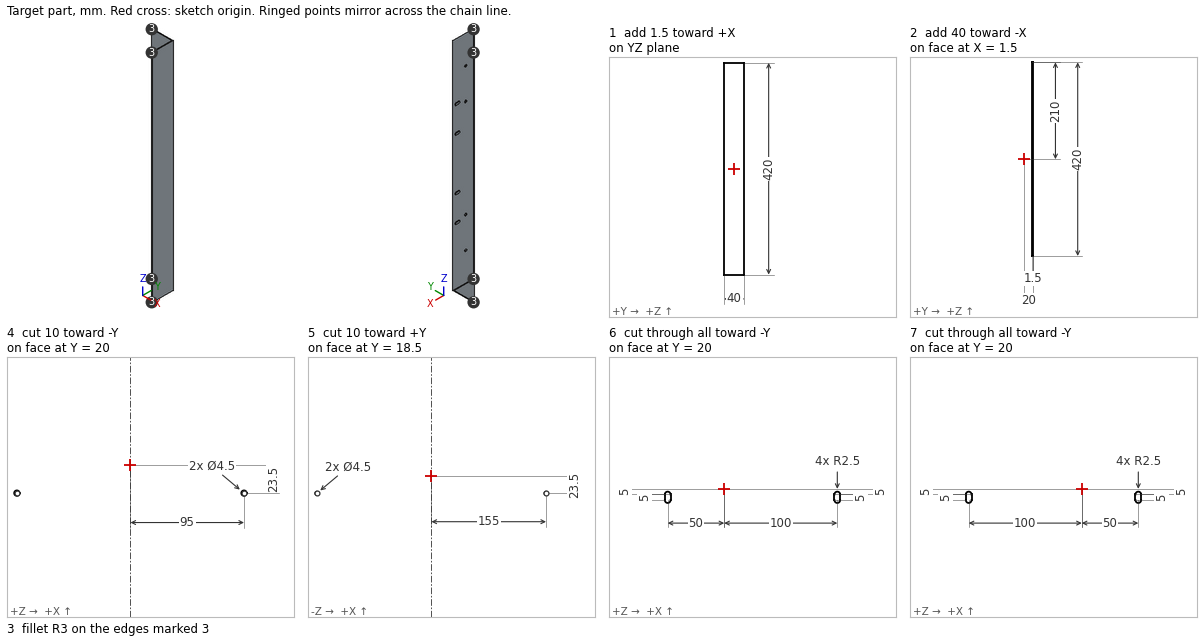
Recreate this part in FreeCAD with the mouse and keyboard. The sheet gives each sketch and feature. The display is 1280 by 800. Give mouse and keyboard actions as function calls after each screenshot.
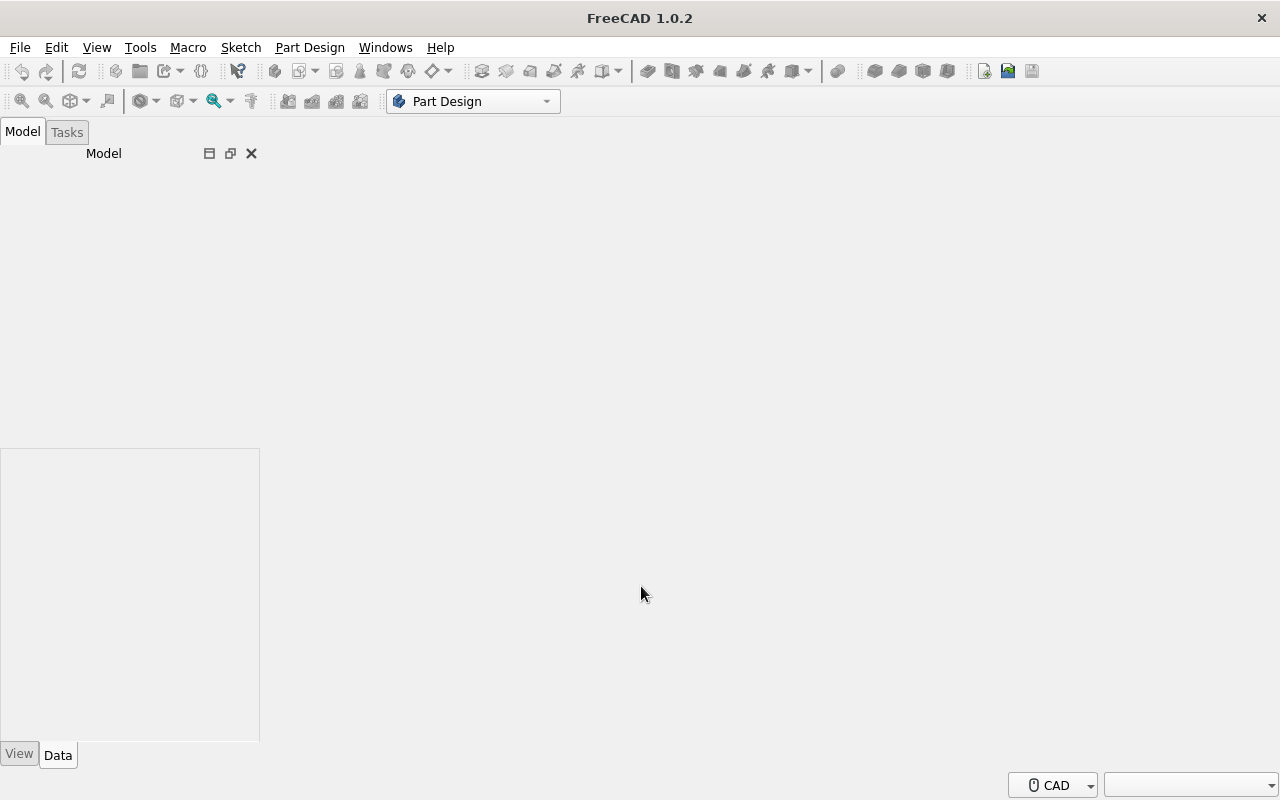
click(984, 72)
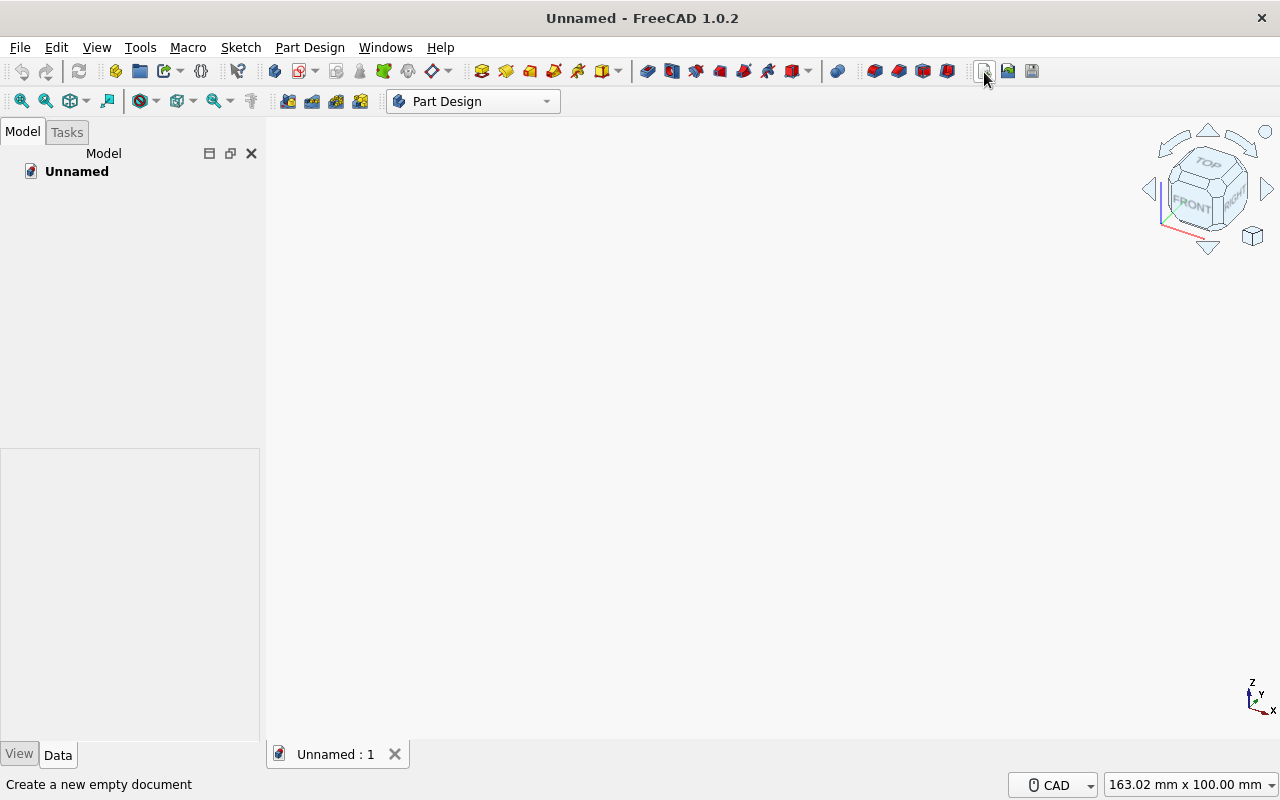
click(300, 72)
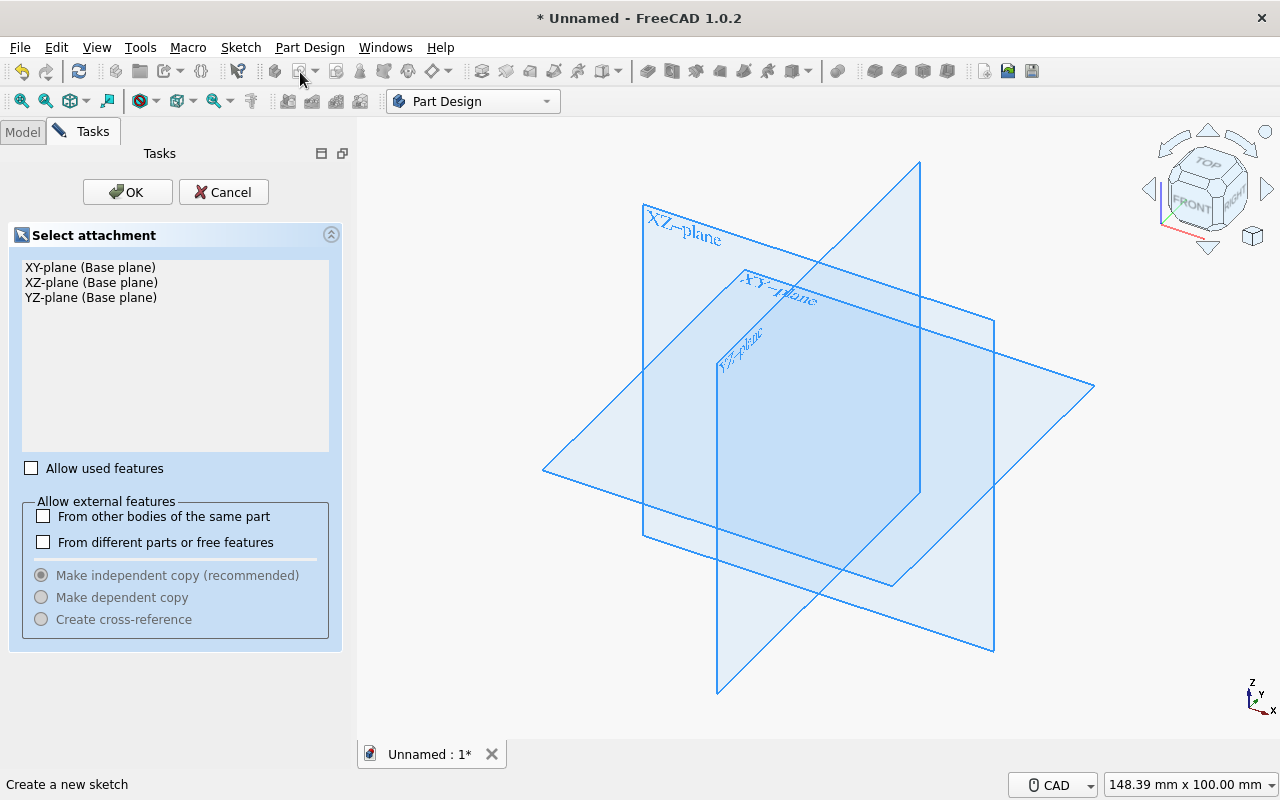
click(82, 298)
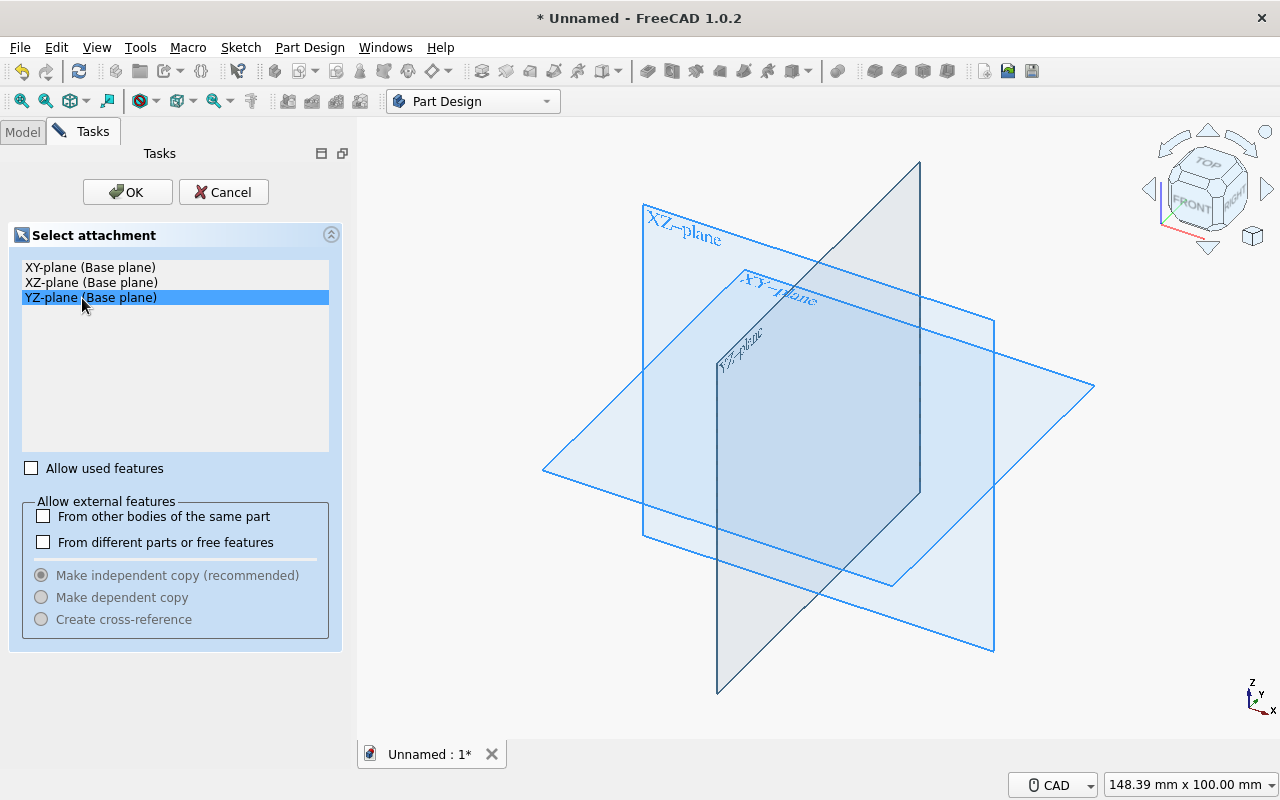
click(128, 192)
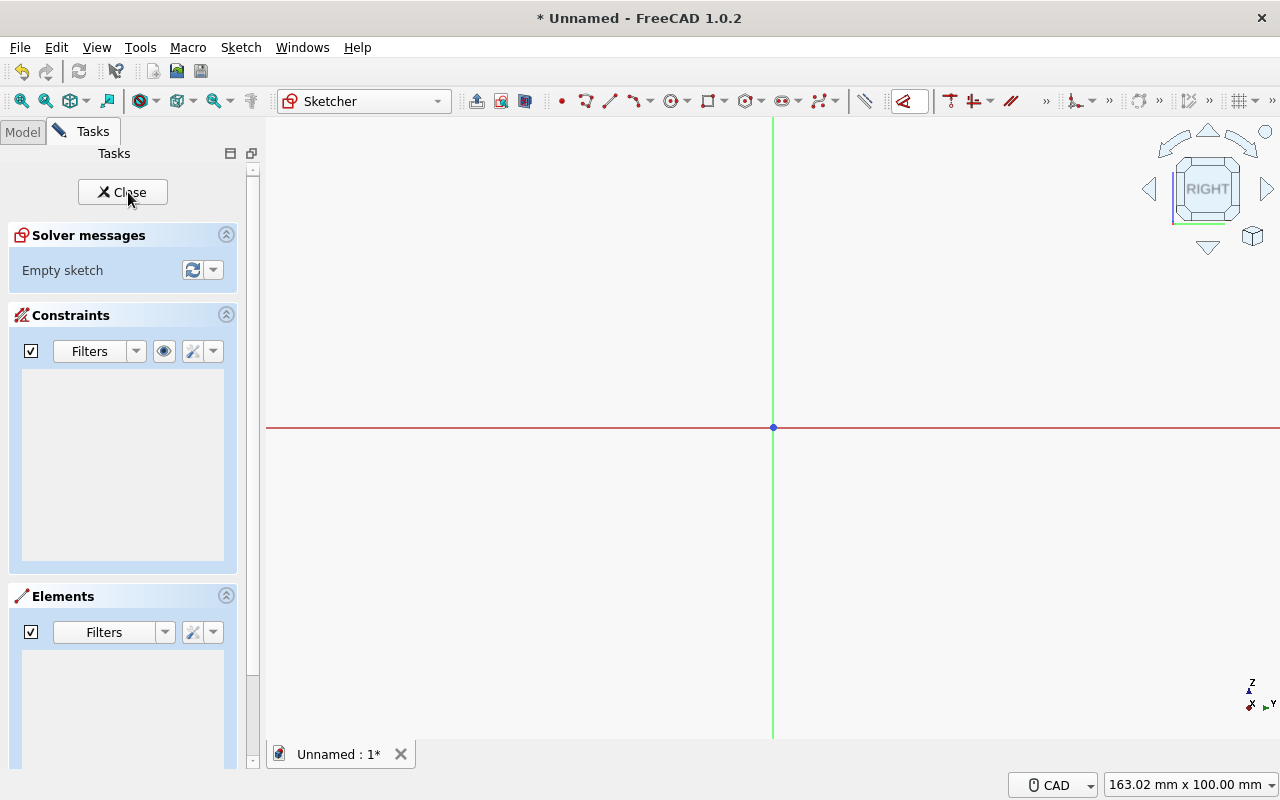
scroll(691, 428, down, 9)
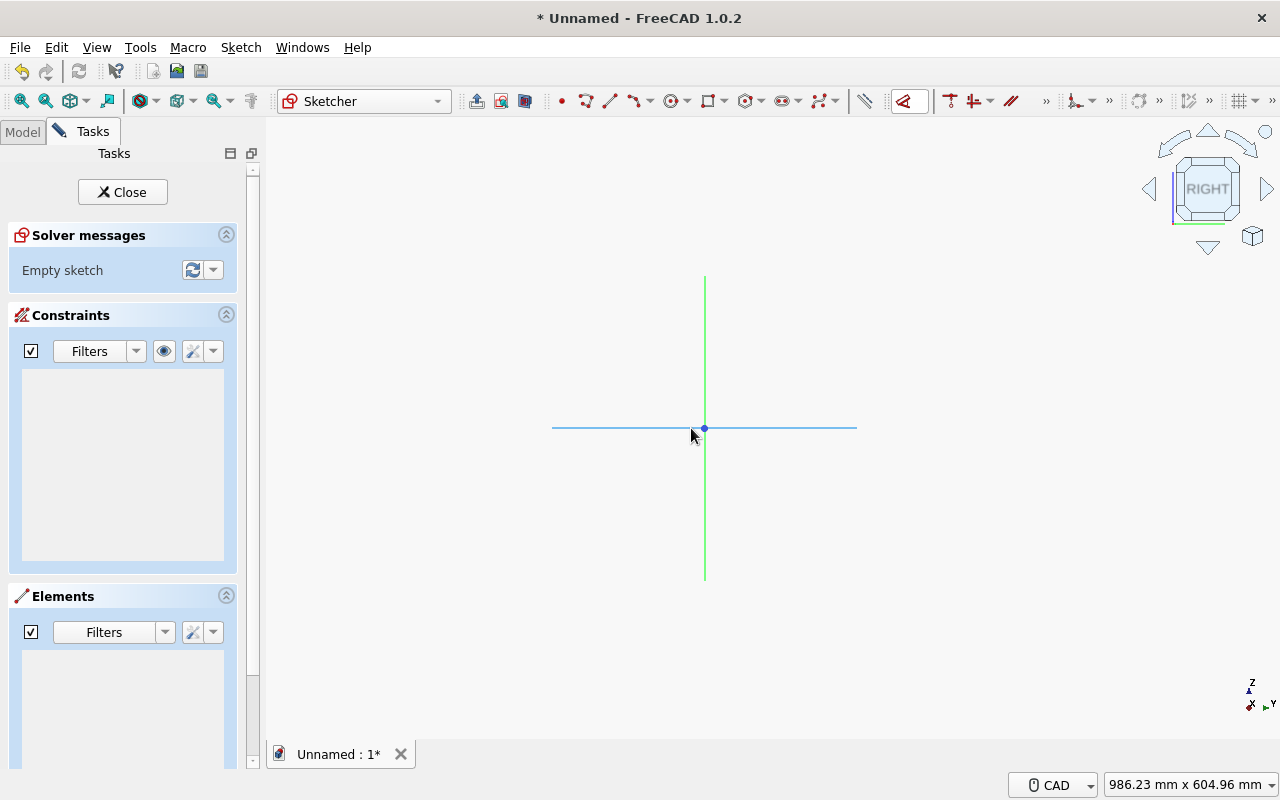
key(g)
key(v)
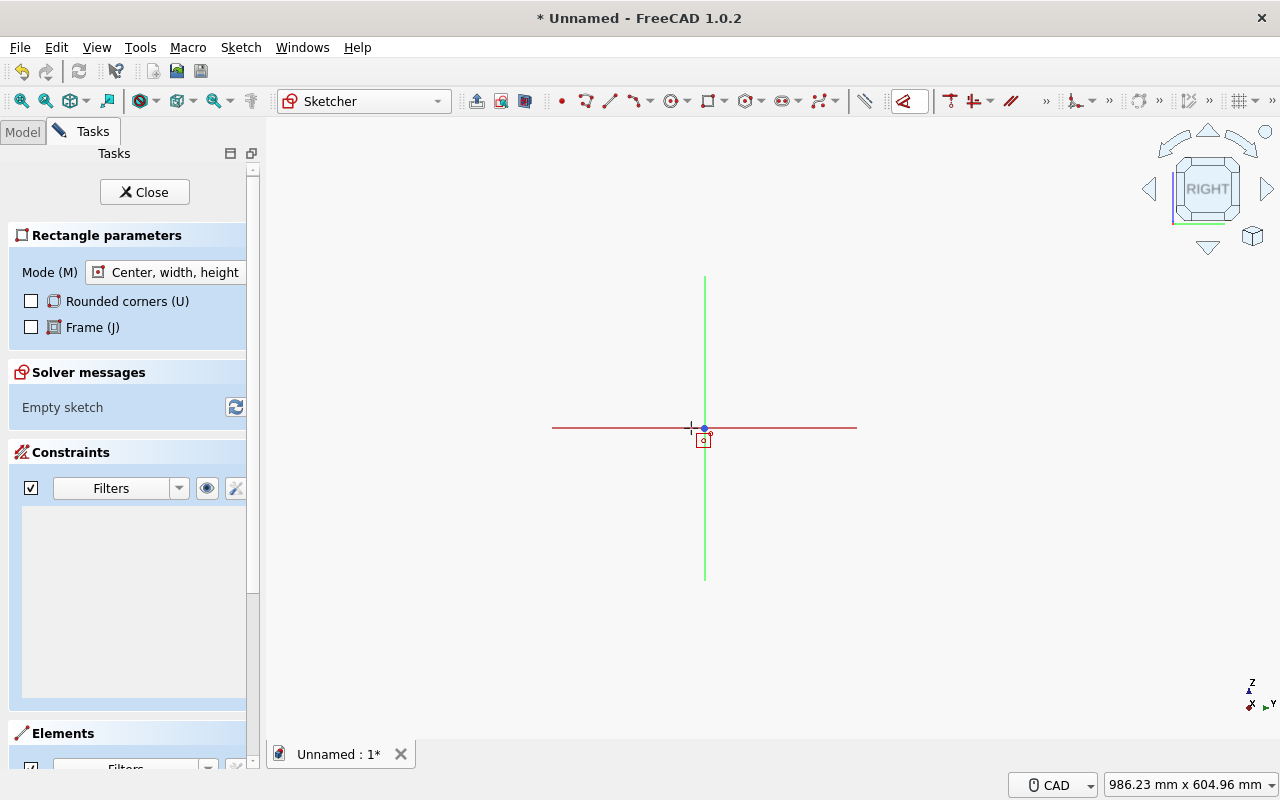
click(705, 428)
click(725, 213)
key(Escape)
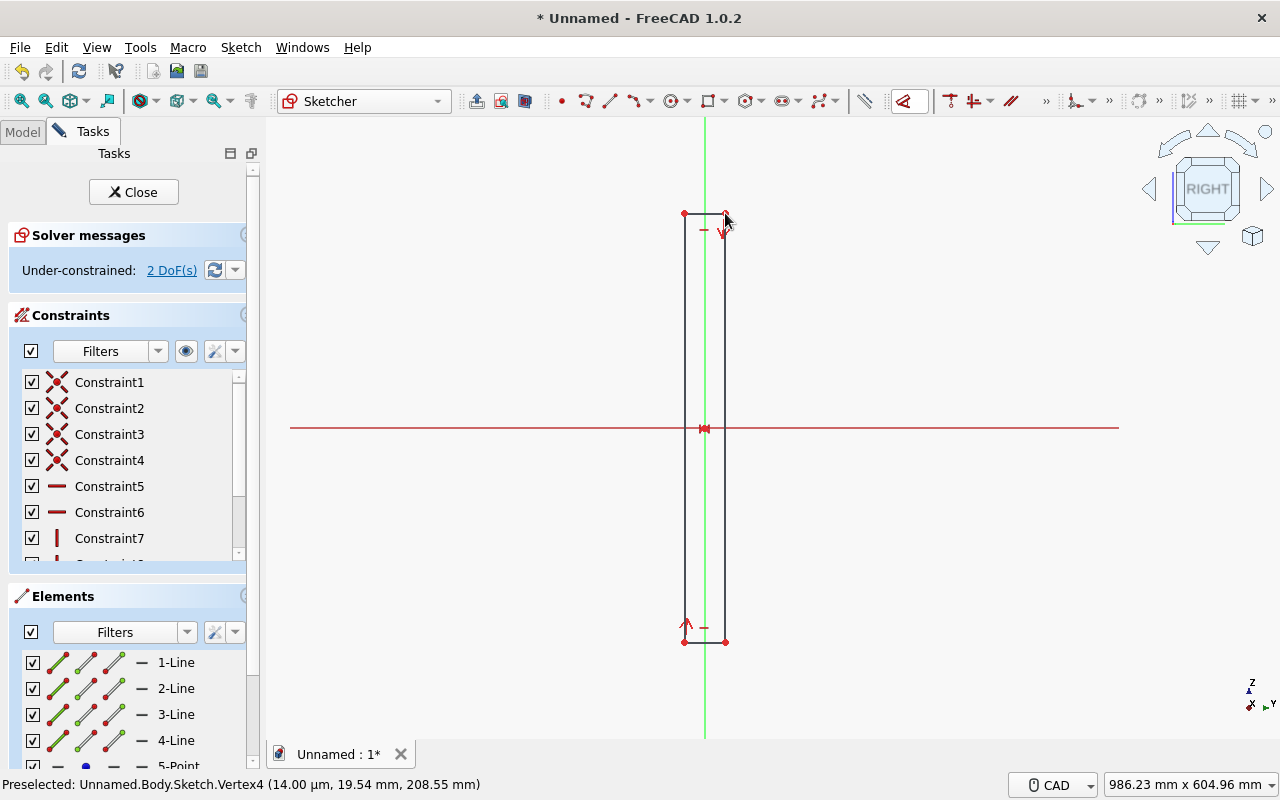
click(904, 102)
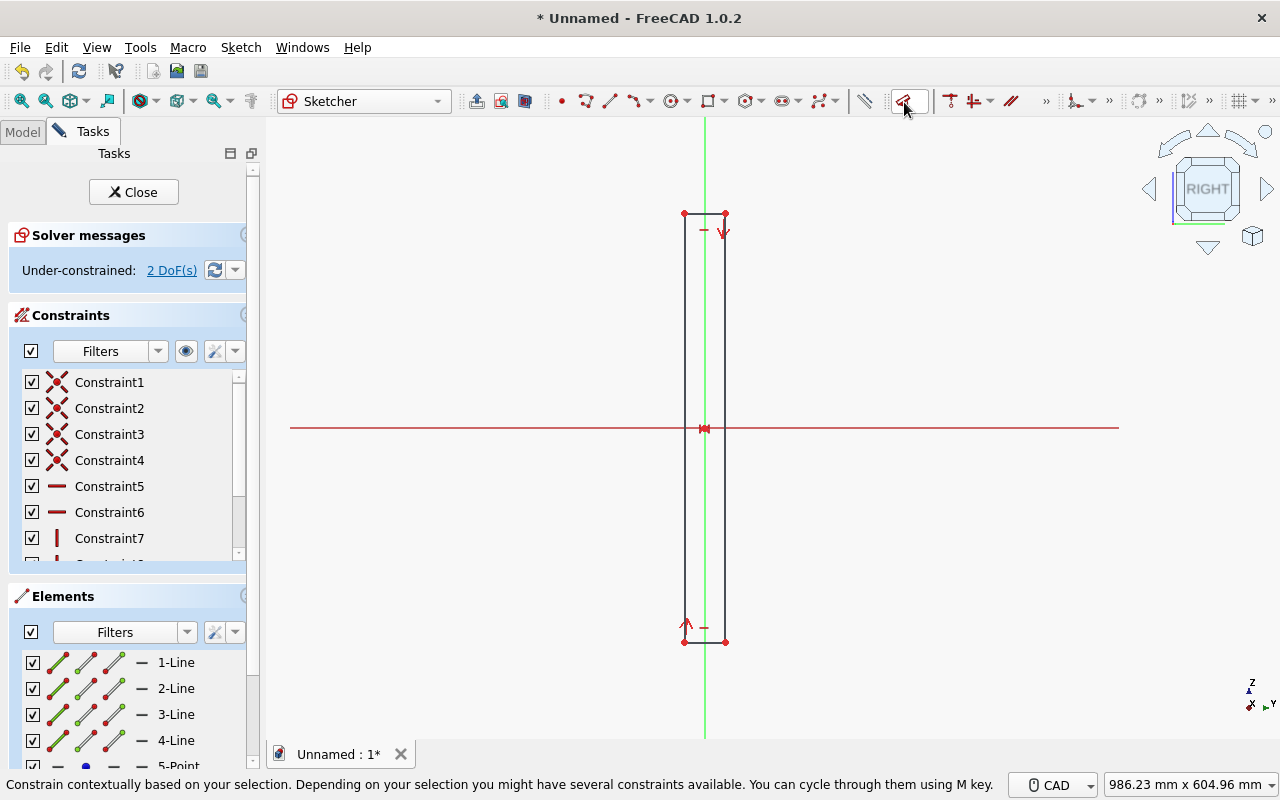
click(705, 643)
click(691, 677)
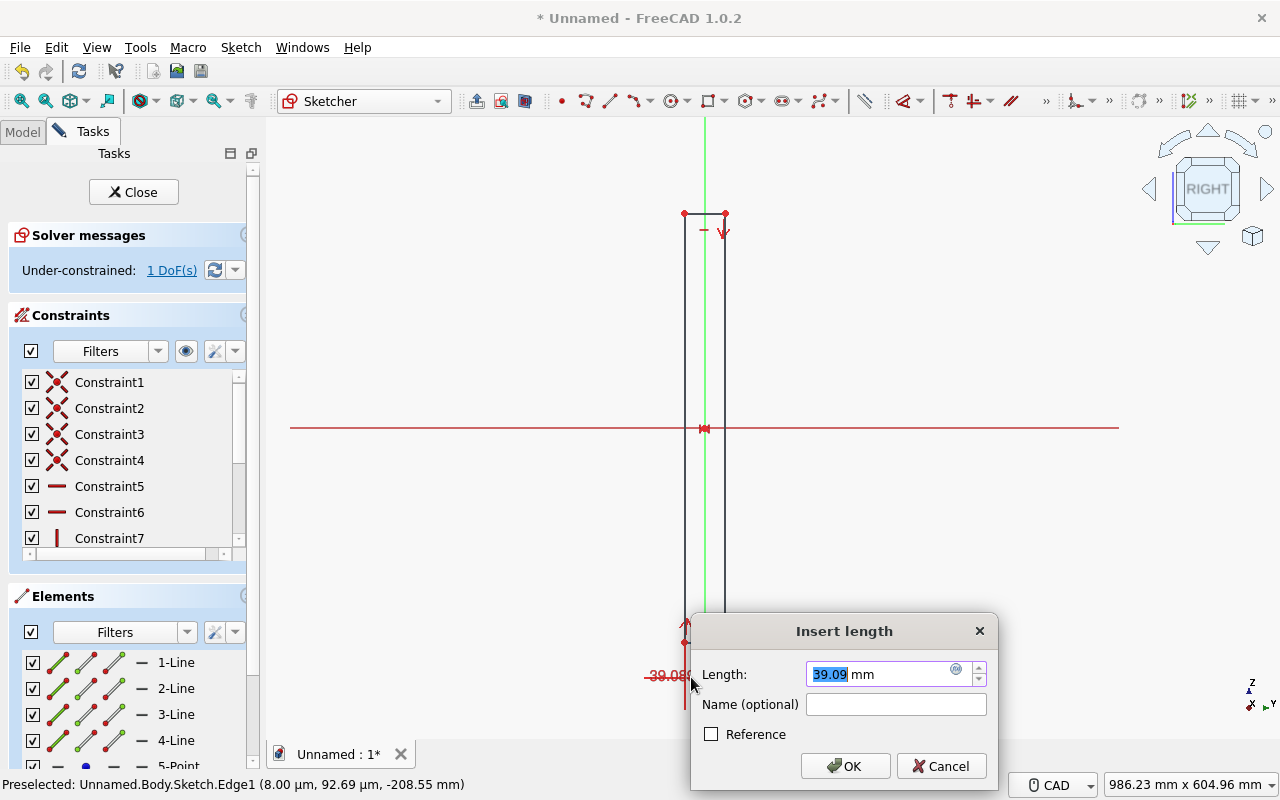
text(40)
key(Return)